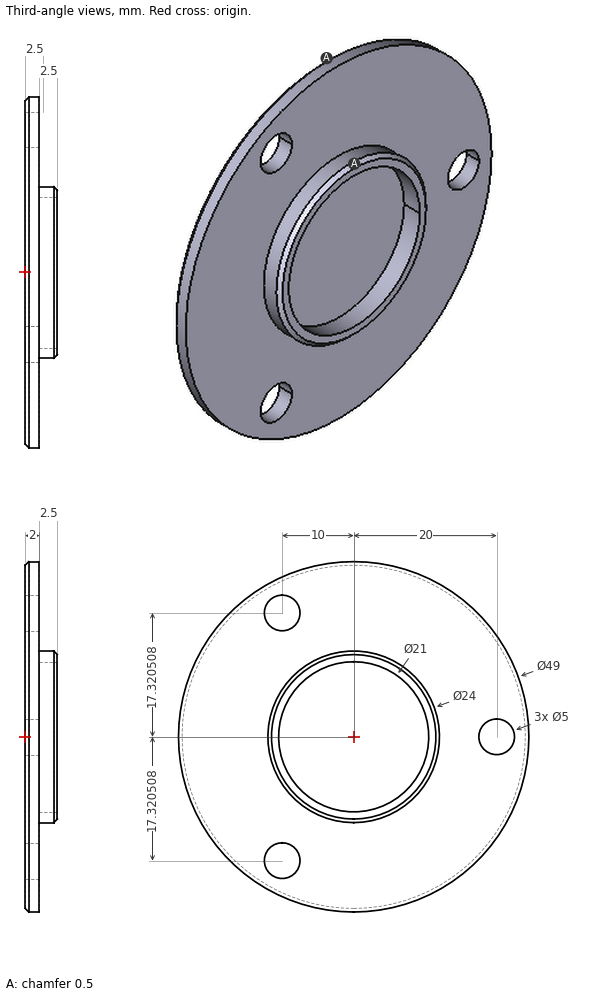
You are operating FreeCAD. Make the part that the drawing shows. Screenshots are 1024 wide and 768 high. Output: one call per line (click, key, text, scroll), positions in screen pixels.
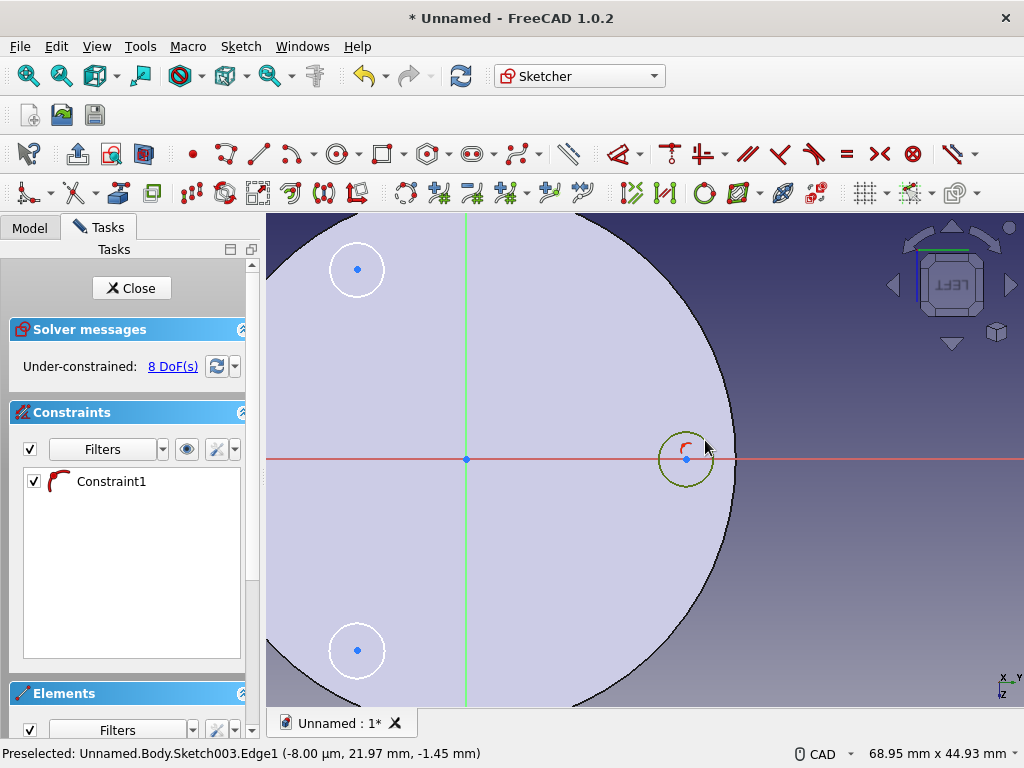
click(376, 631)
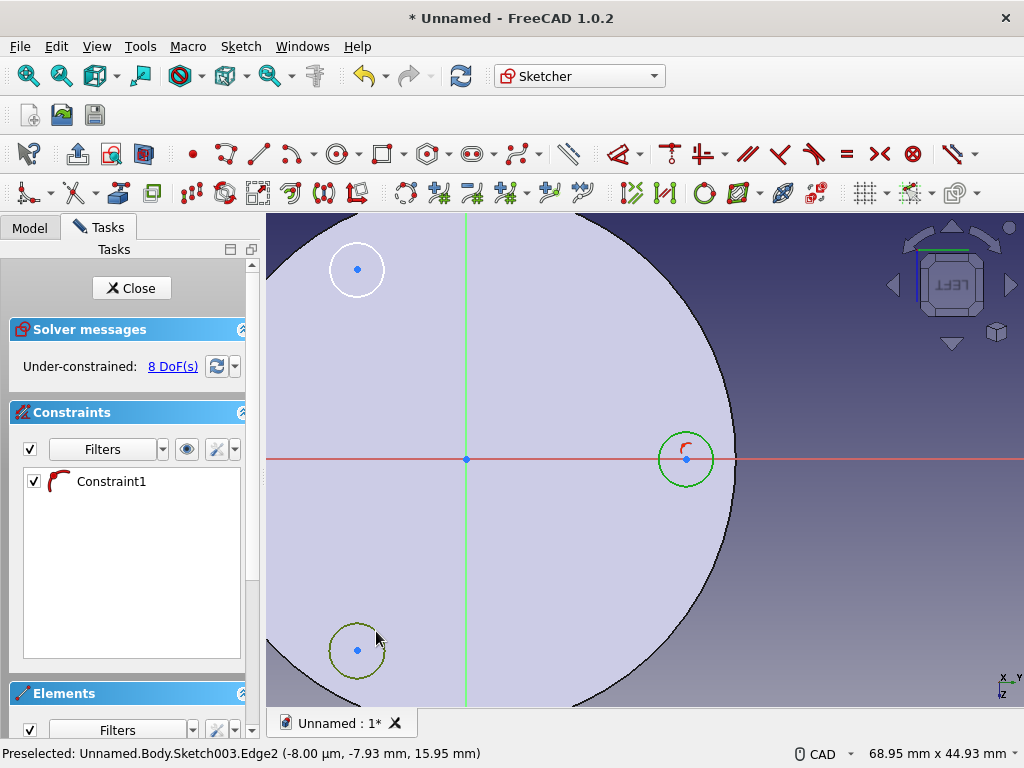
click(376, 251)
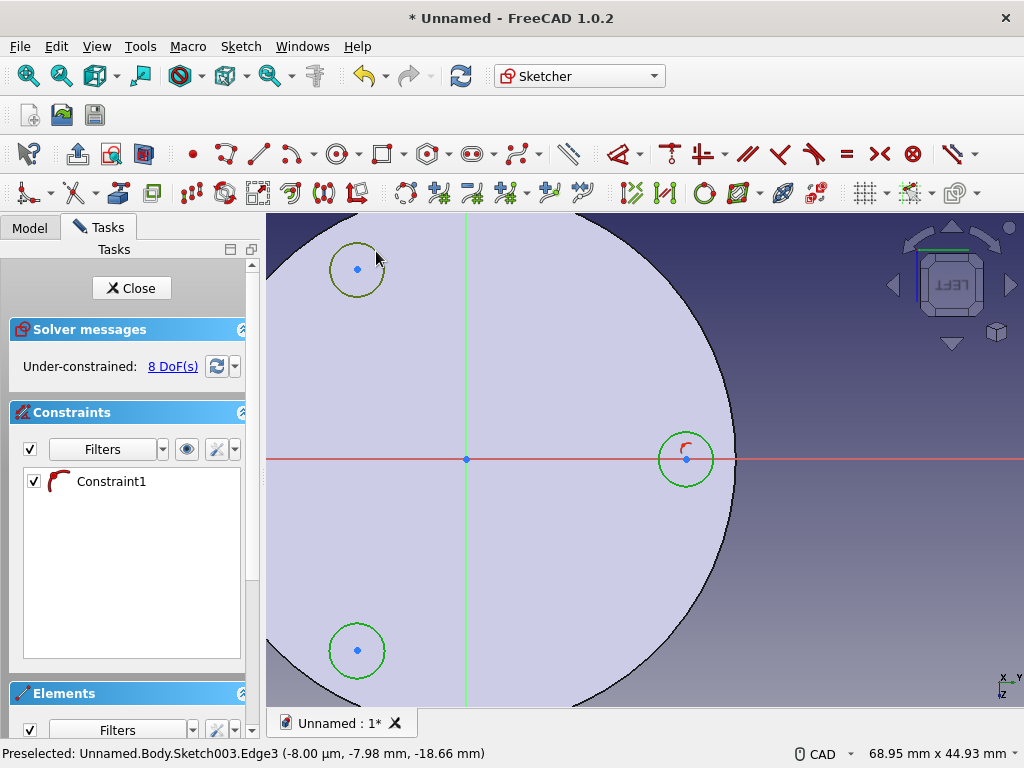
click(847, 154)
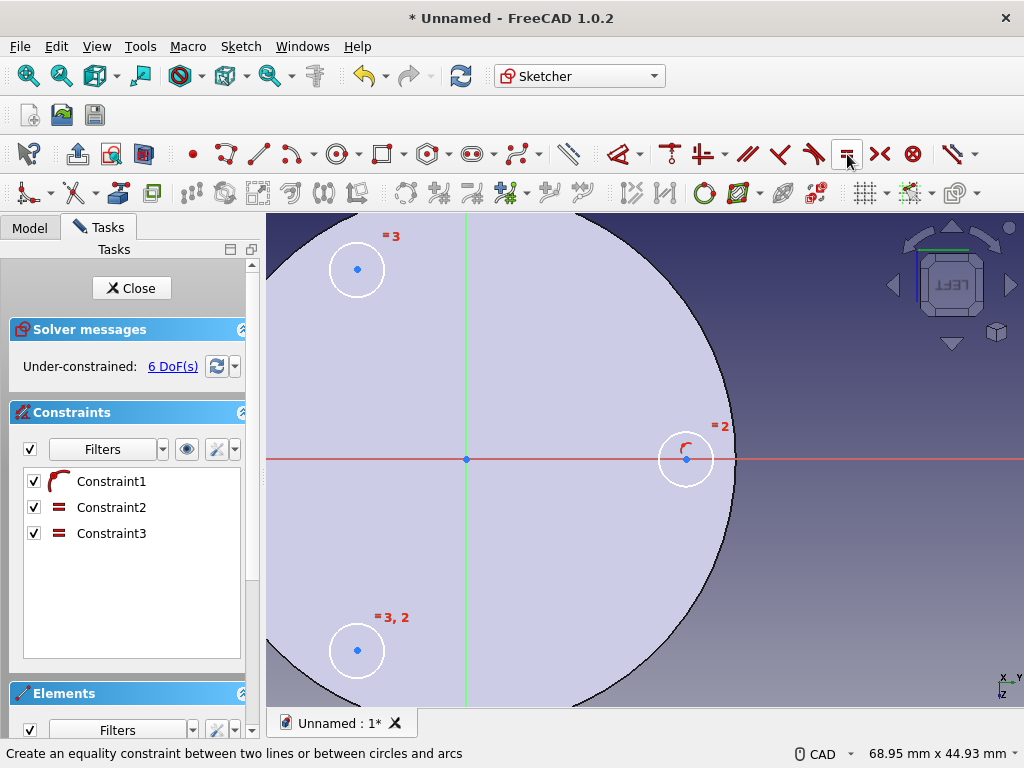
click(357, 651)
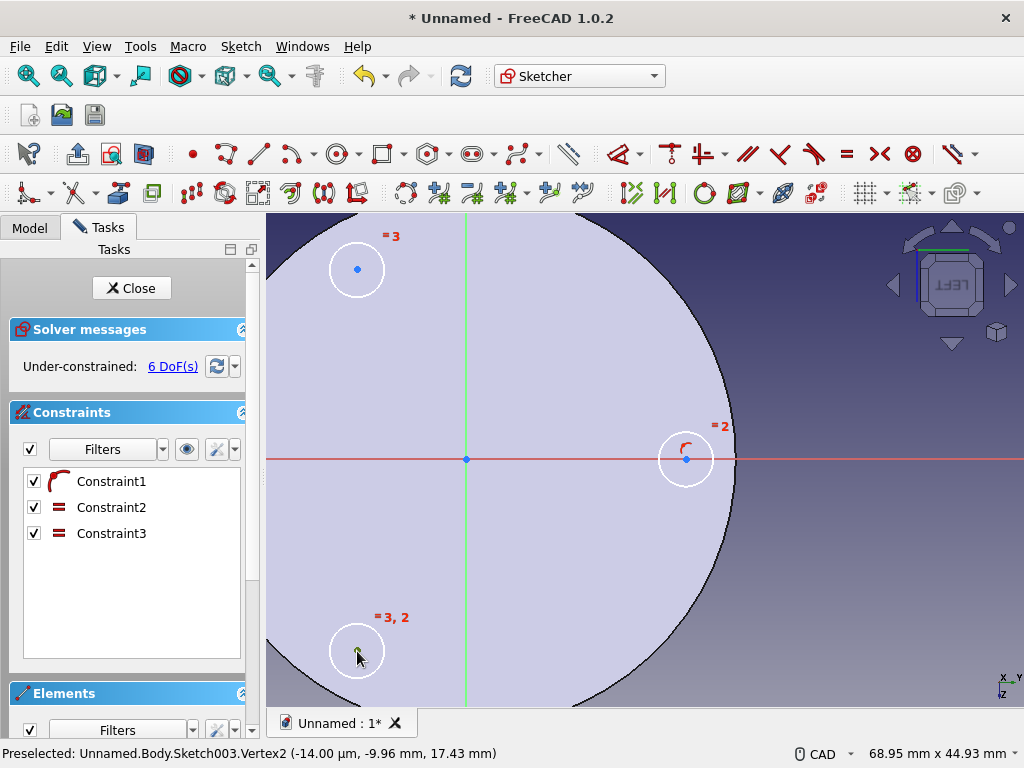
click(357, 270)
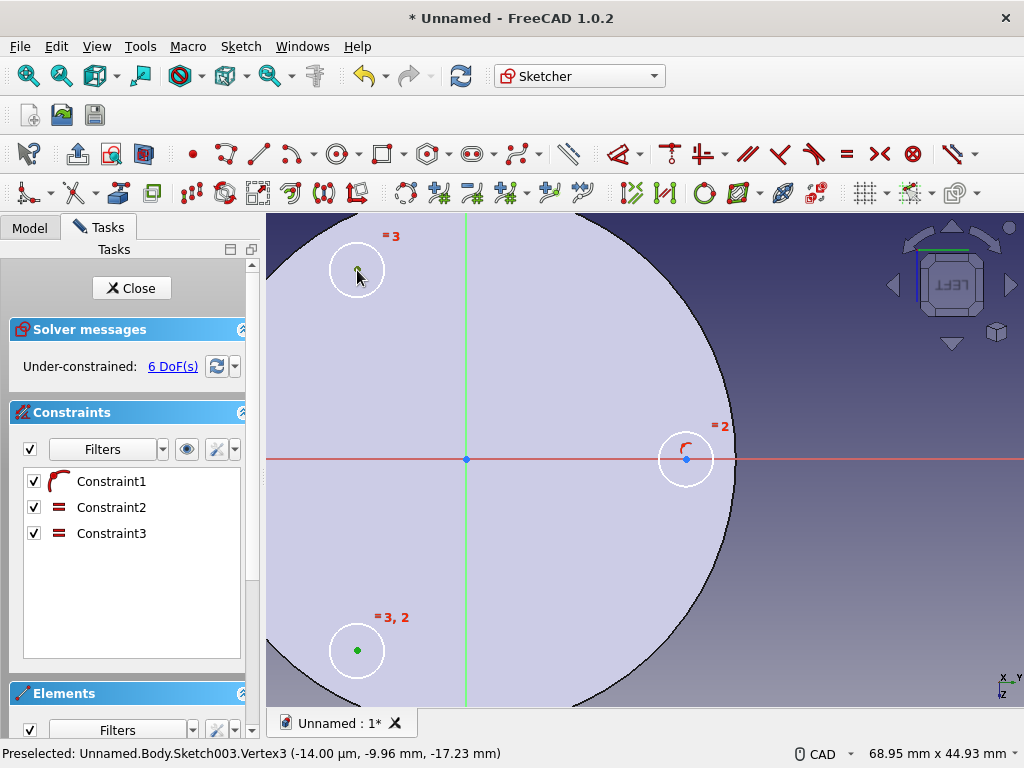
key(v)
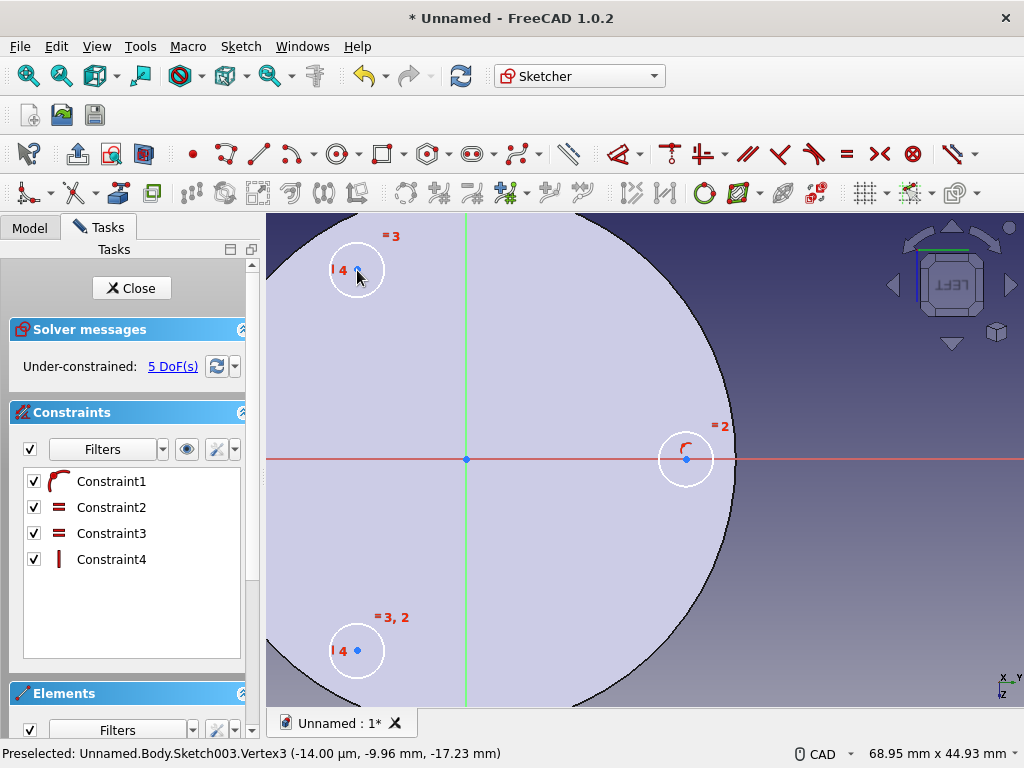
click(618, 154)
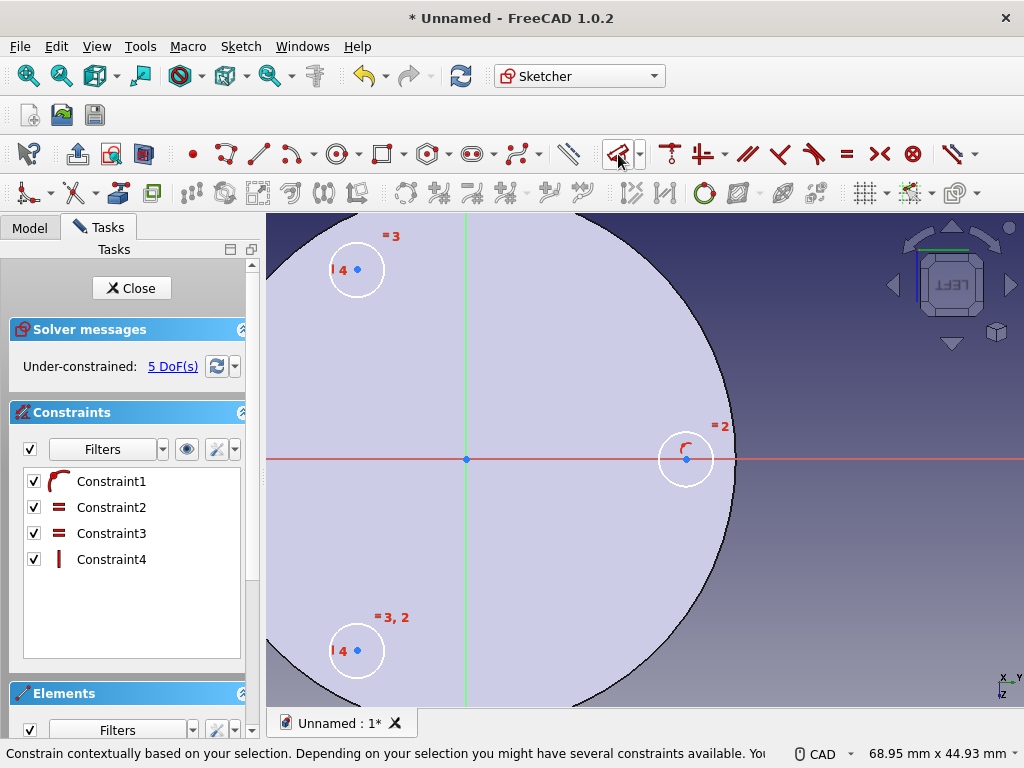
click(705, 440)
click(727, 417)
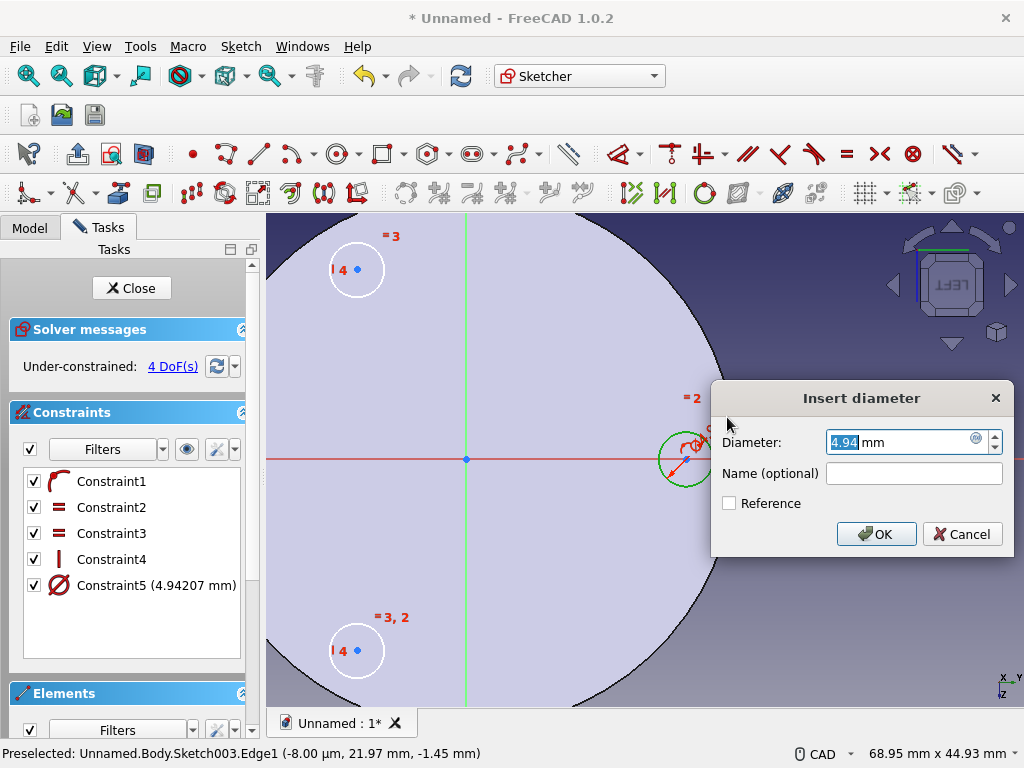
text(5)
key(Return)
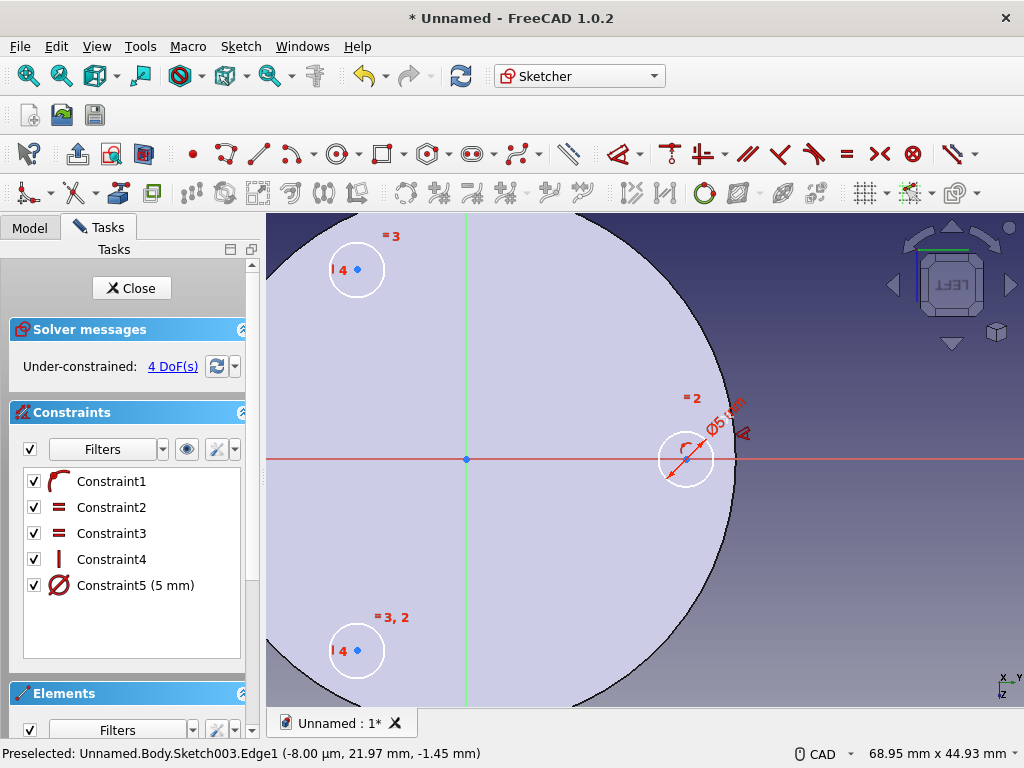
click(686, 459)
click(576, 493)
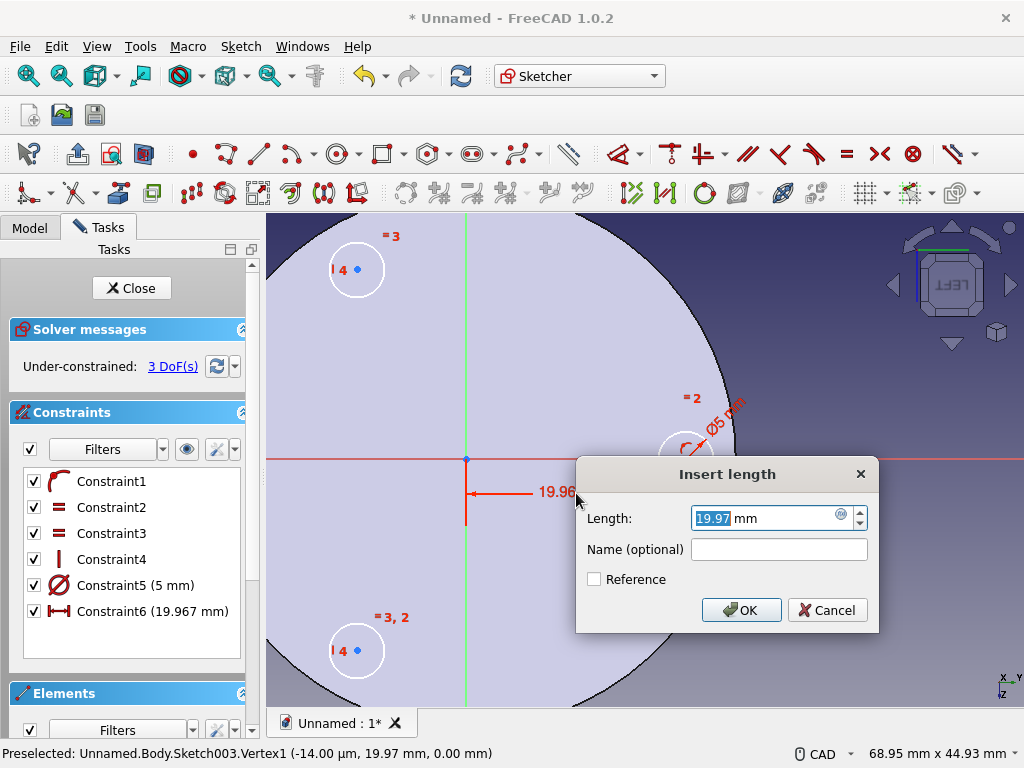
text(20)
key(Return)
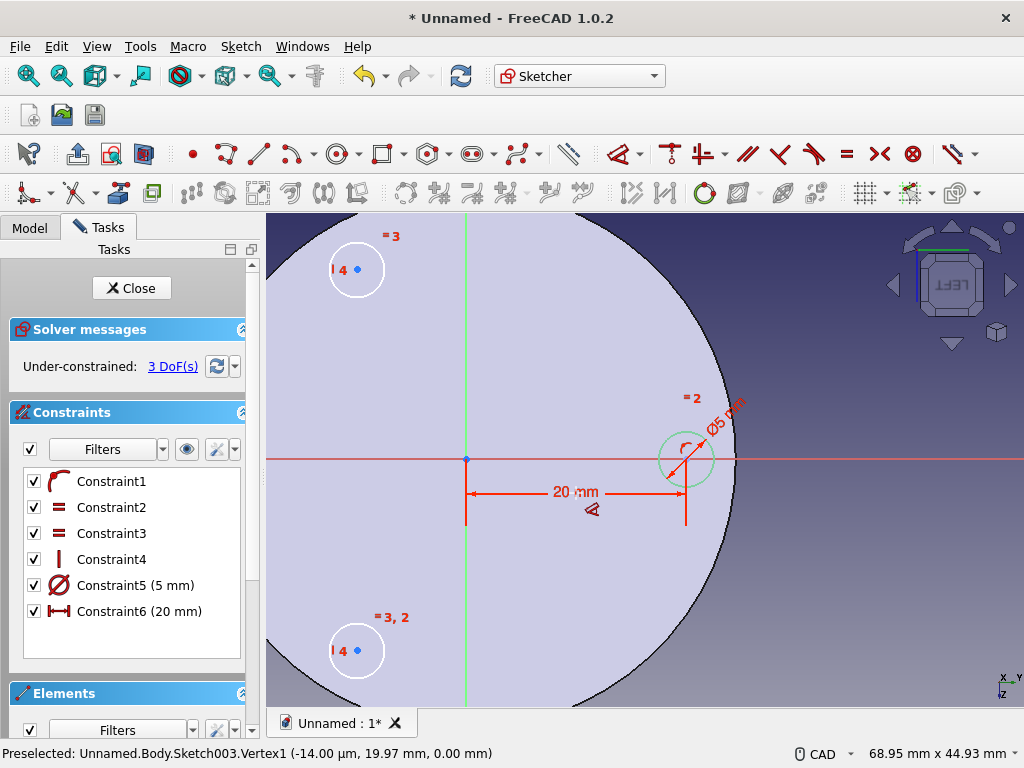
click(357, 651)
click(412, 425)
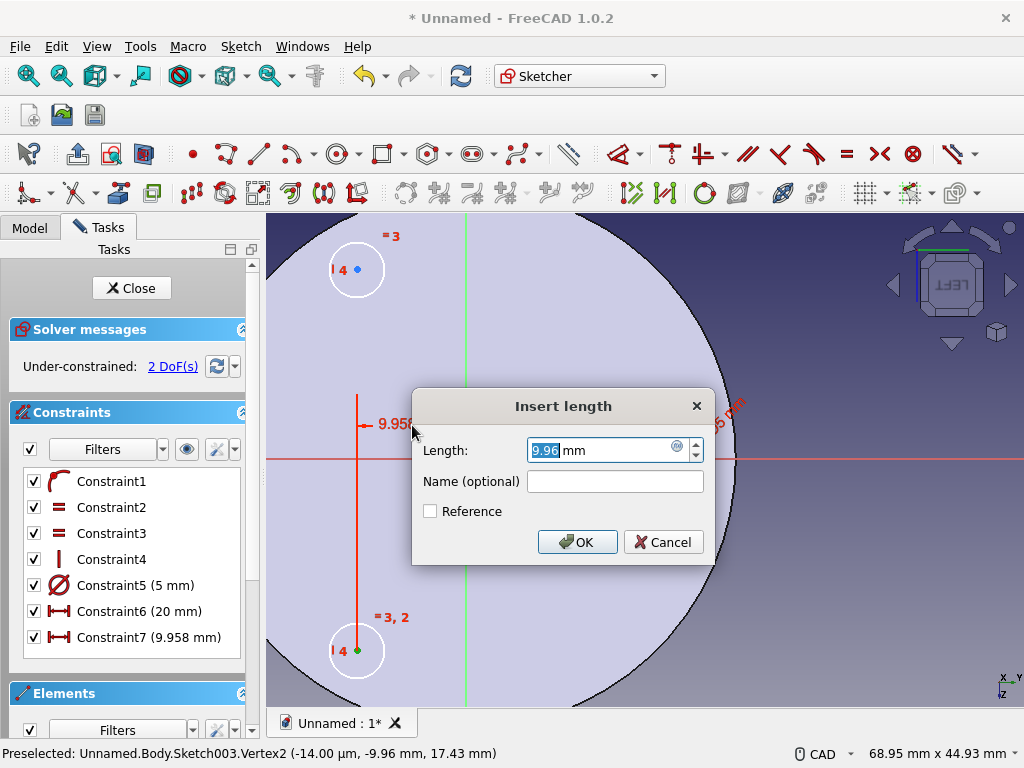
text(10)
key(Return)